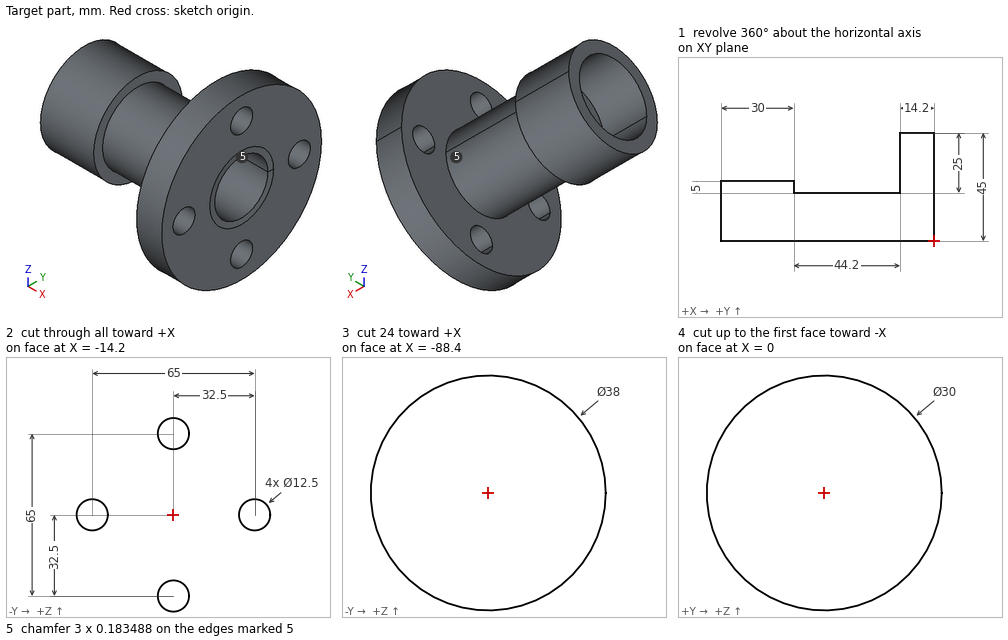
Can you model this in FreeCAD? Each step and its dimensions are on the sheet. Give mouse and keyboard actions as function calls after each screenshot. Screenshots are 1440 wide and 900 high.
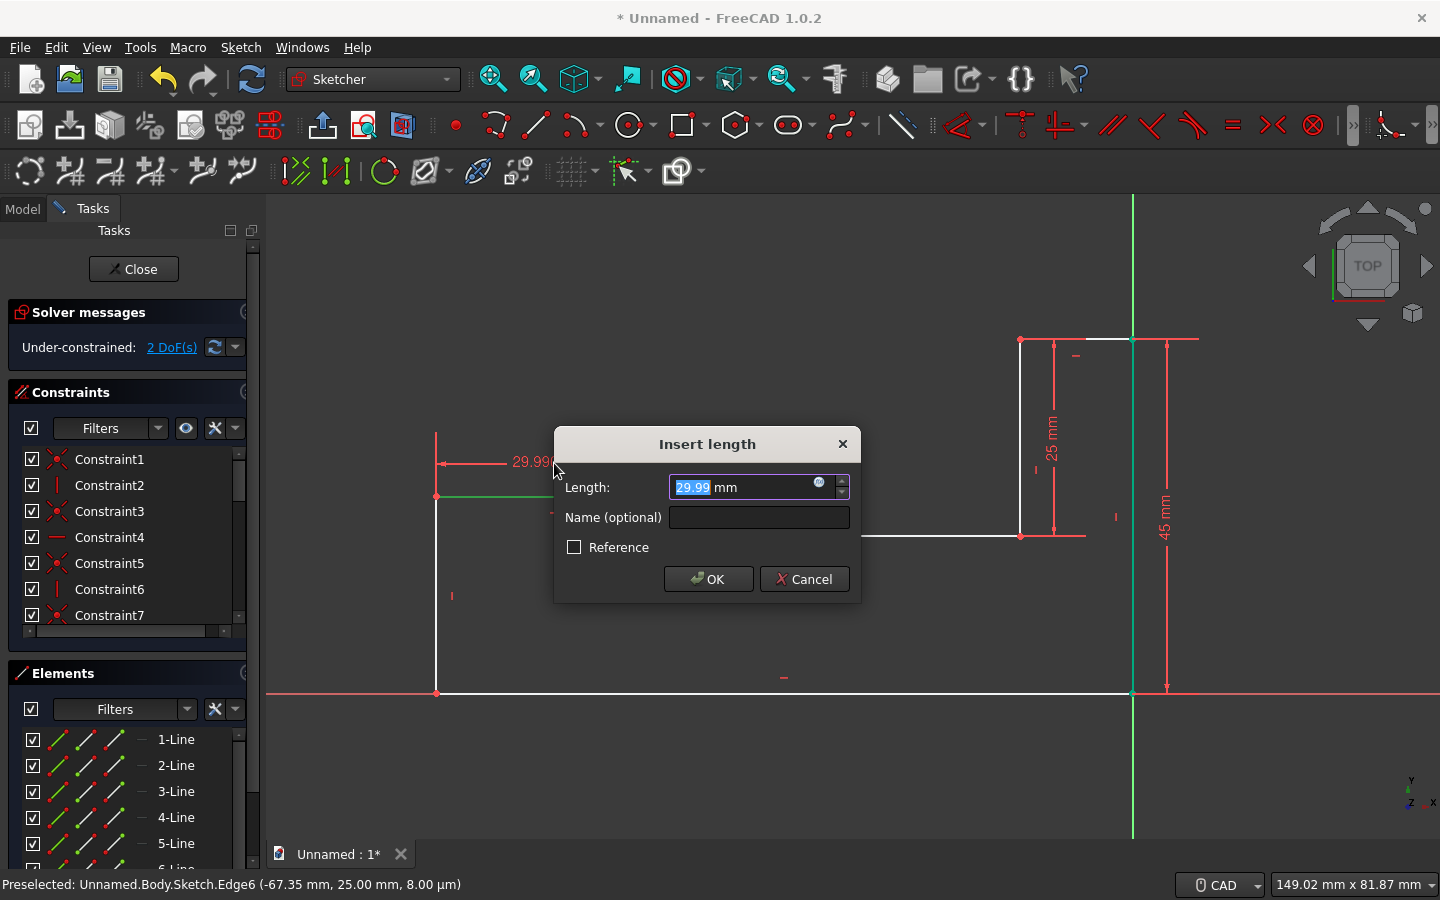
text(30)
key(Return)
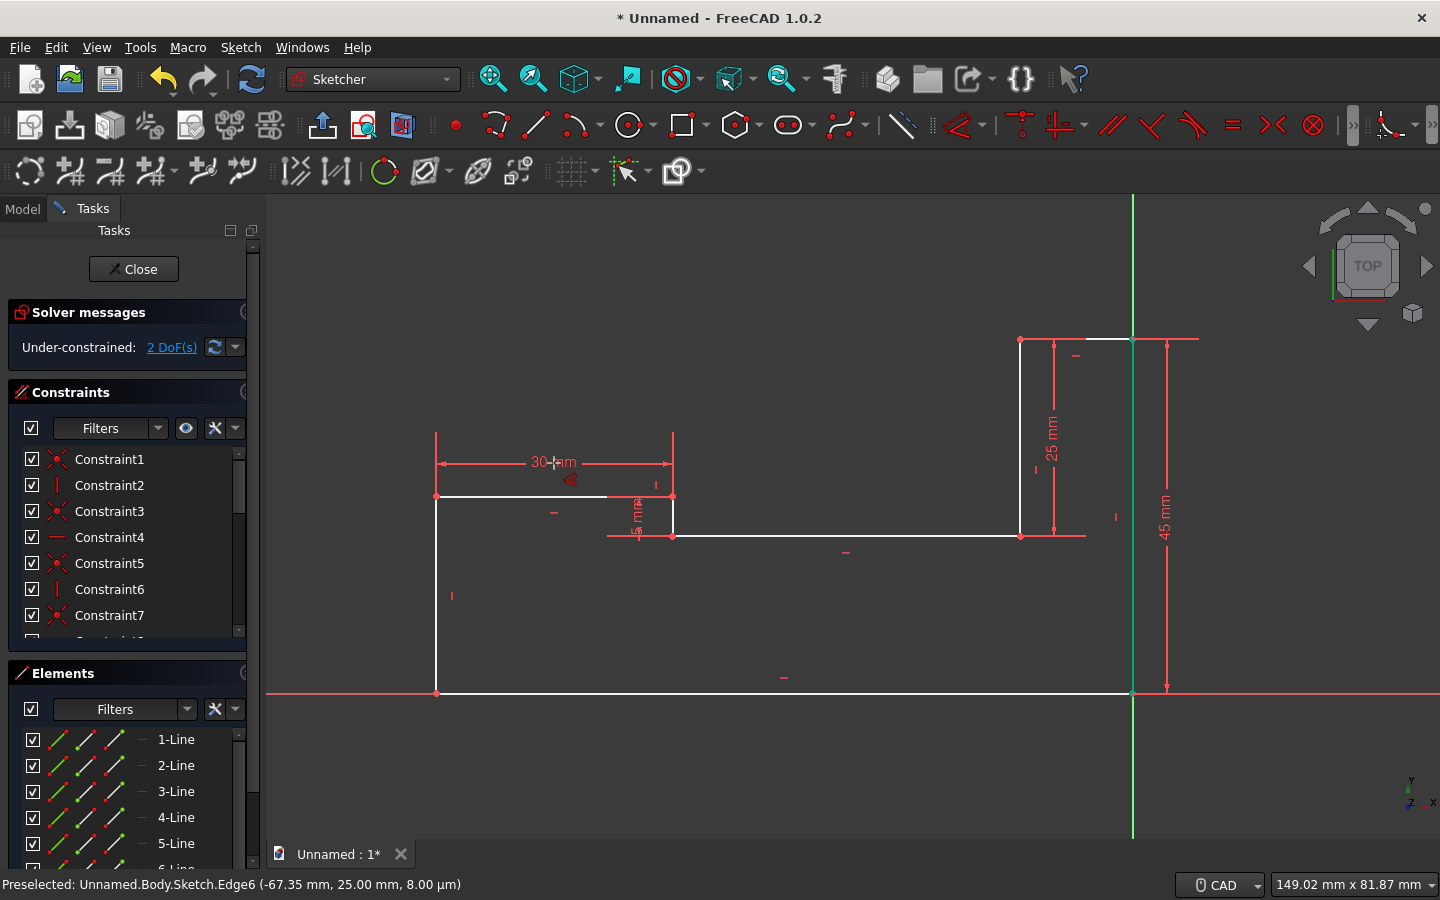
click(1099, 339)
click(1077, 305)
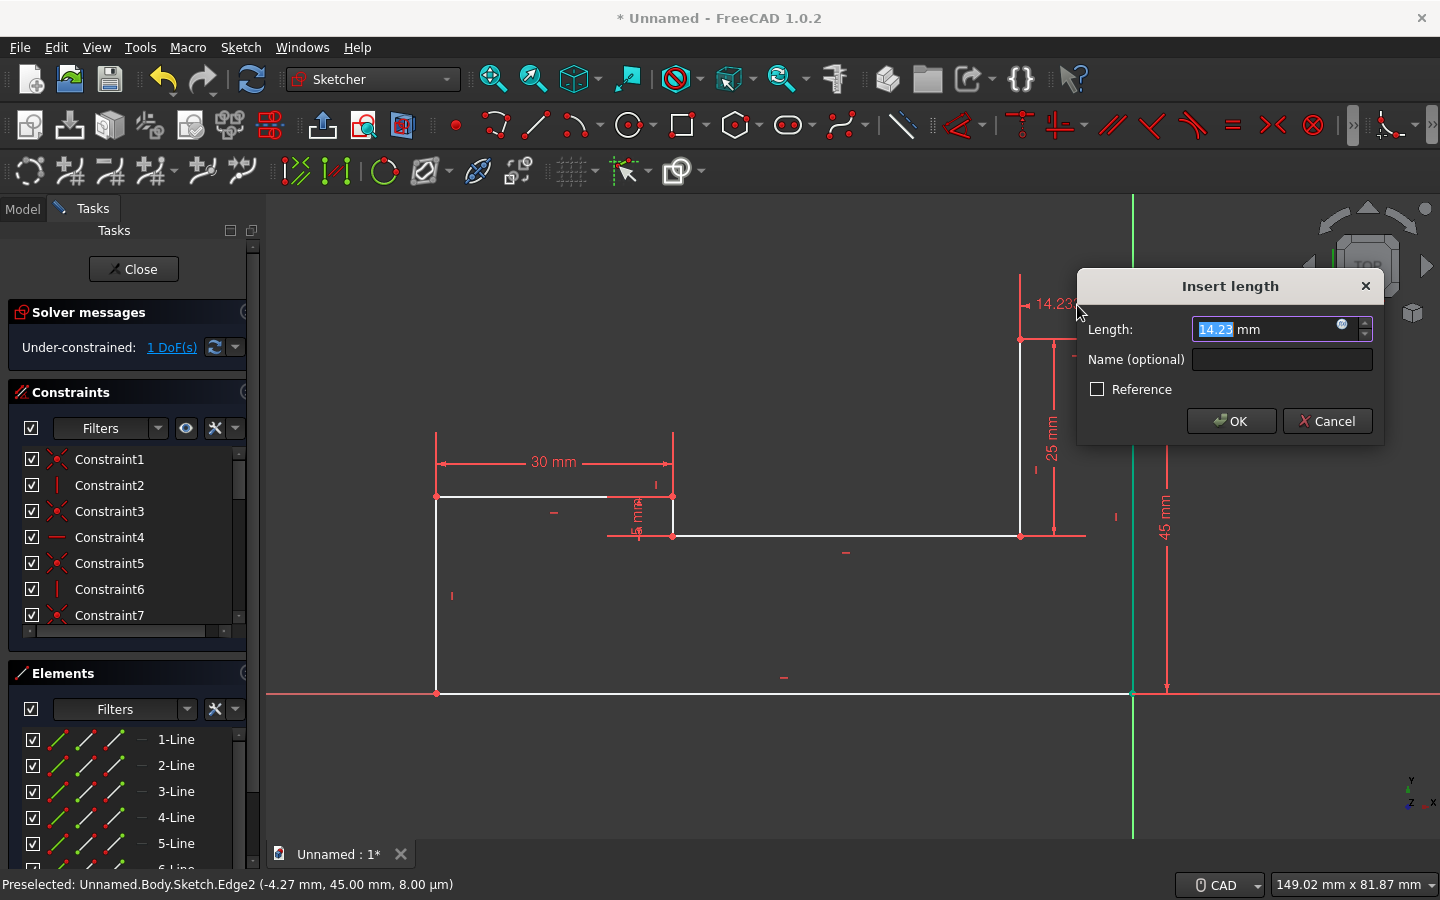
text(14.2)
key(Return)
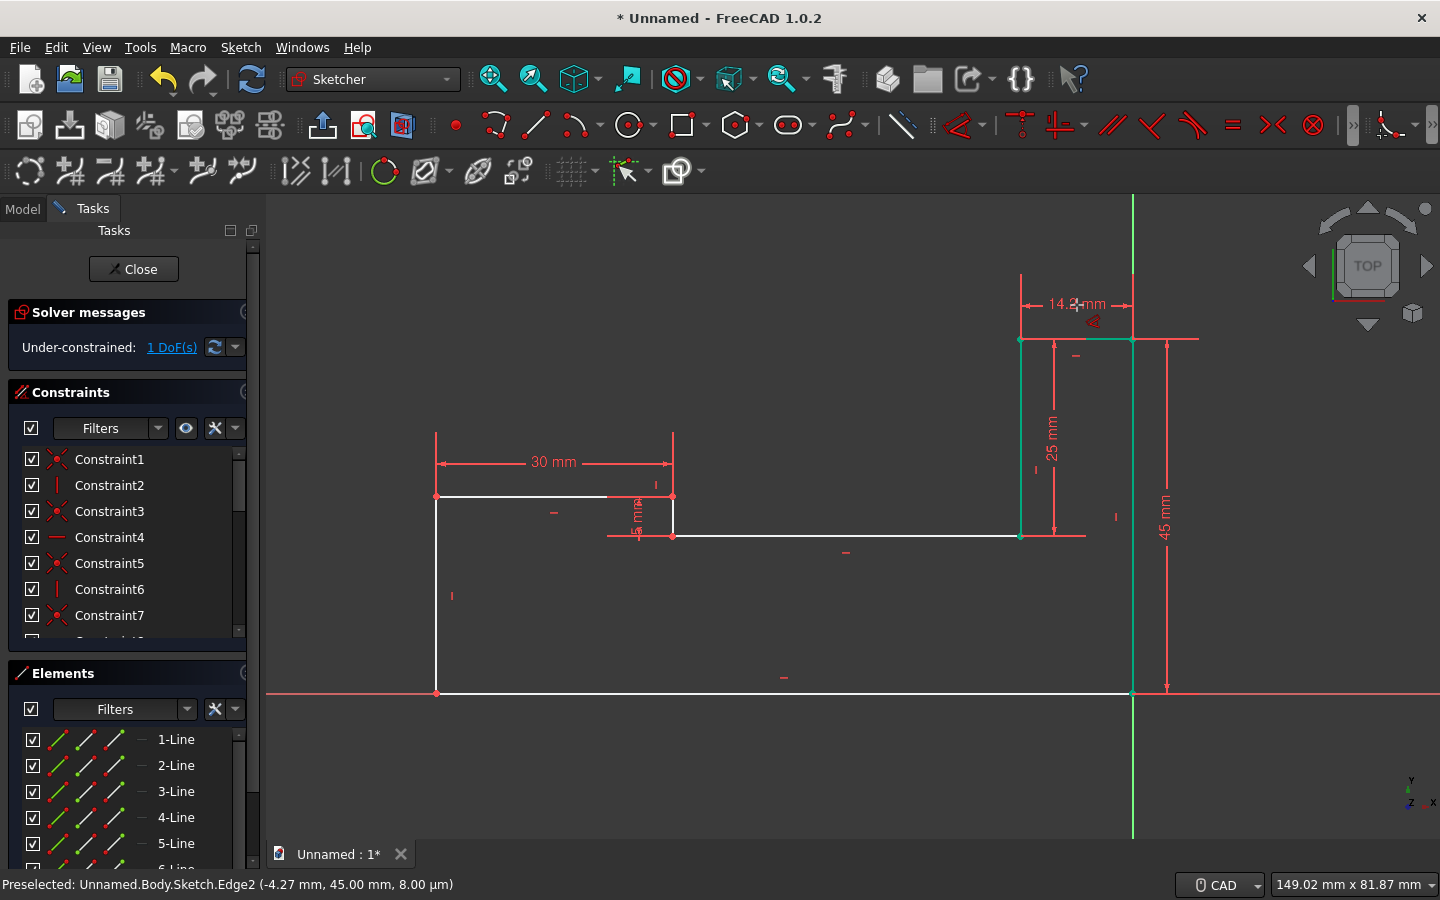
click(916, 536)
click(847, 570)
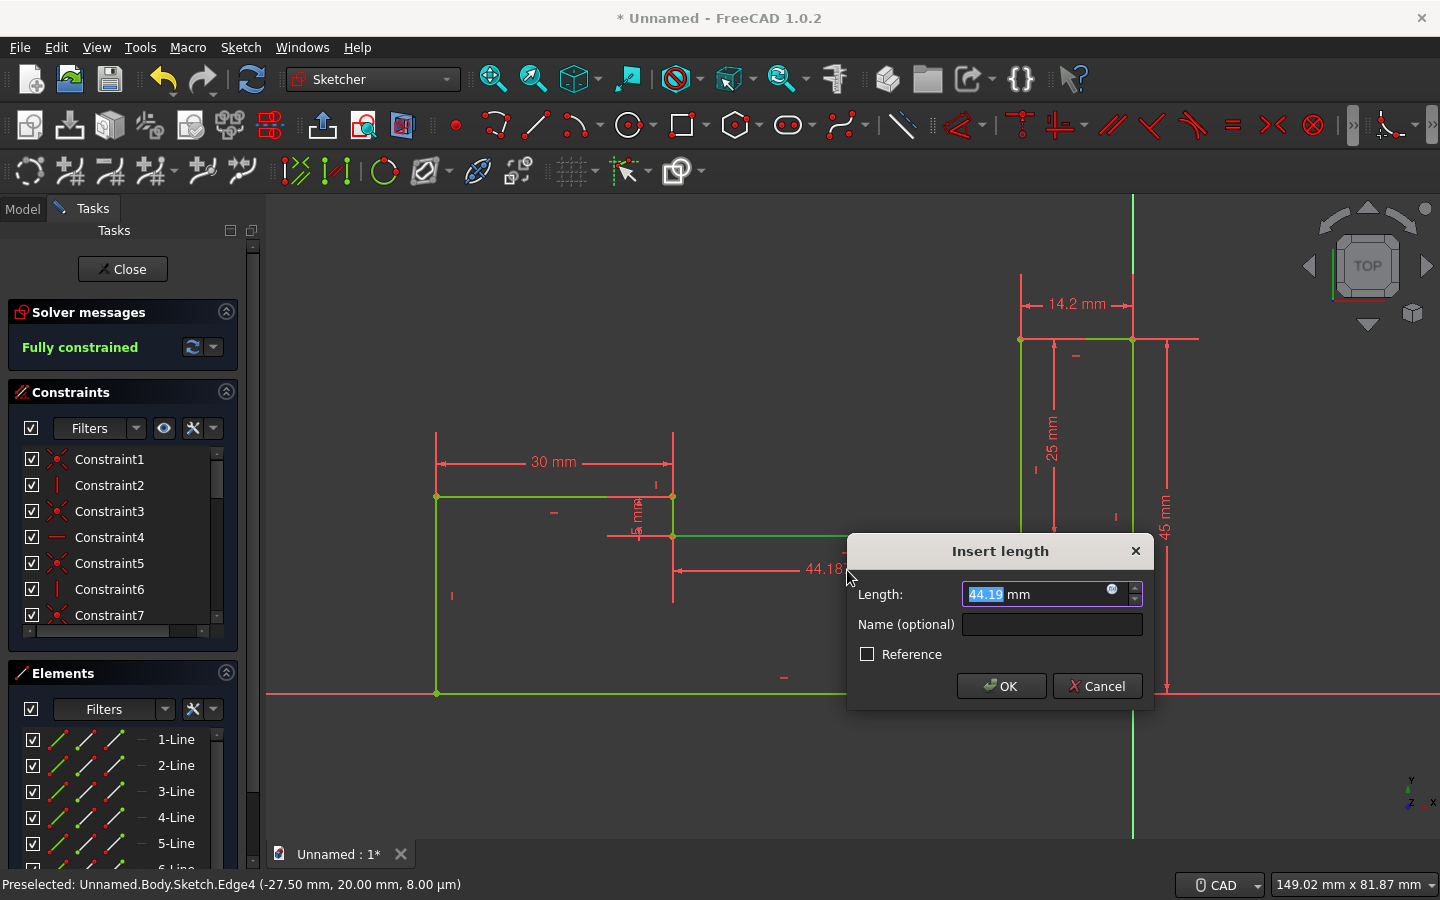
text(44.2)
key(Return)
key(Escape)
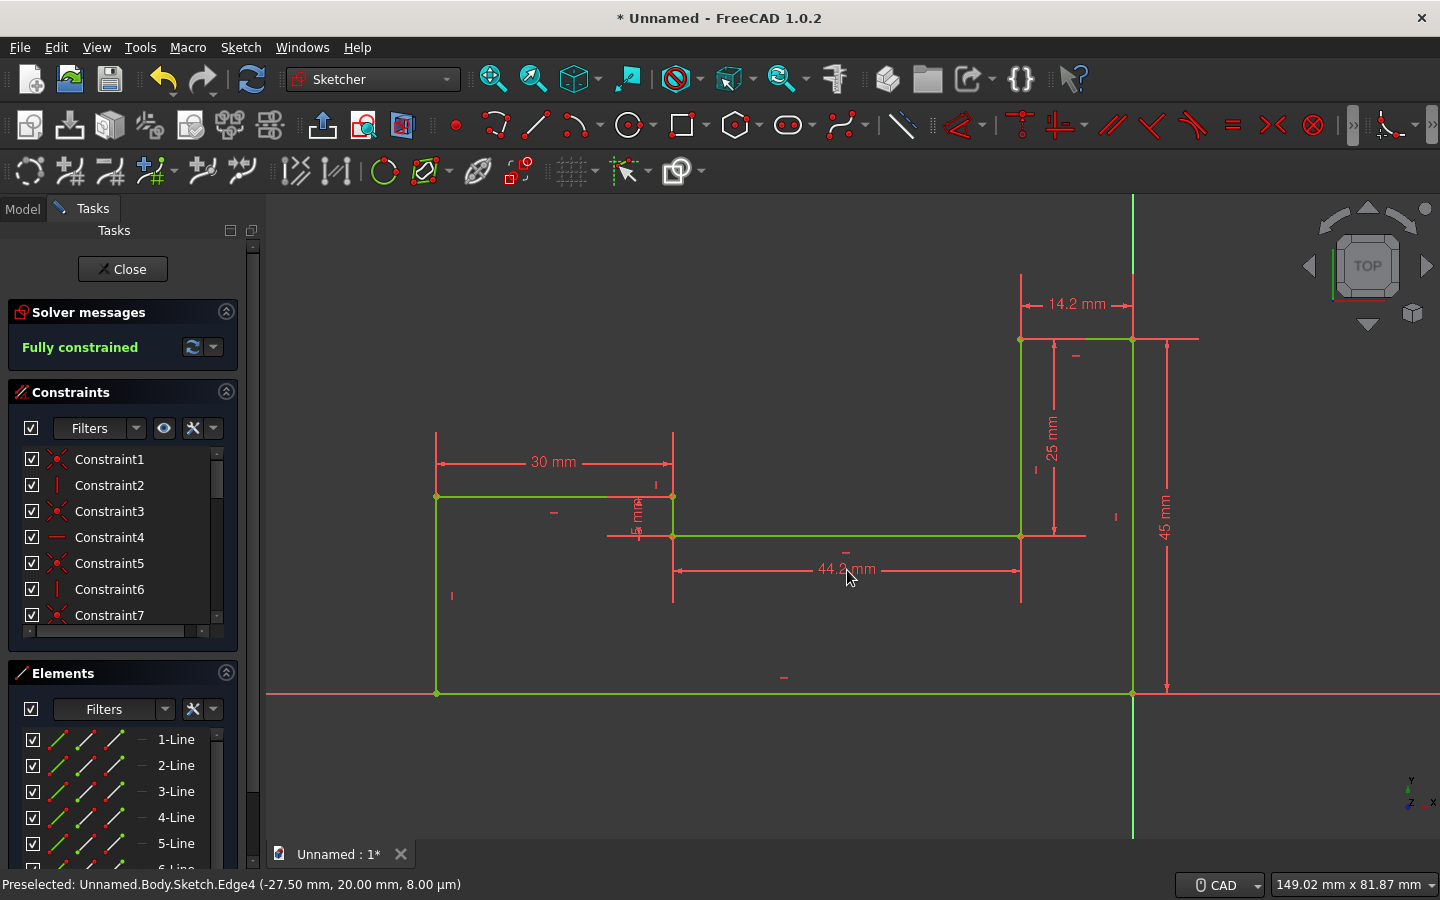
click(123, 269)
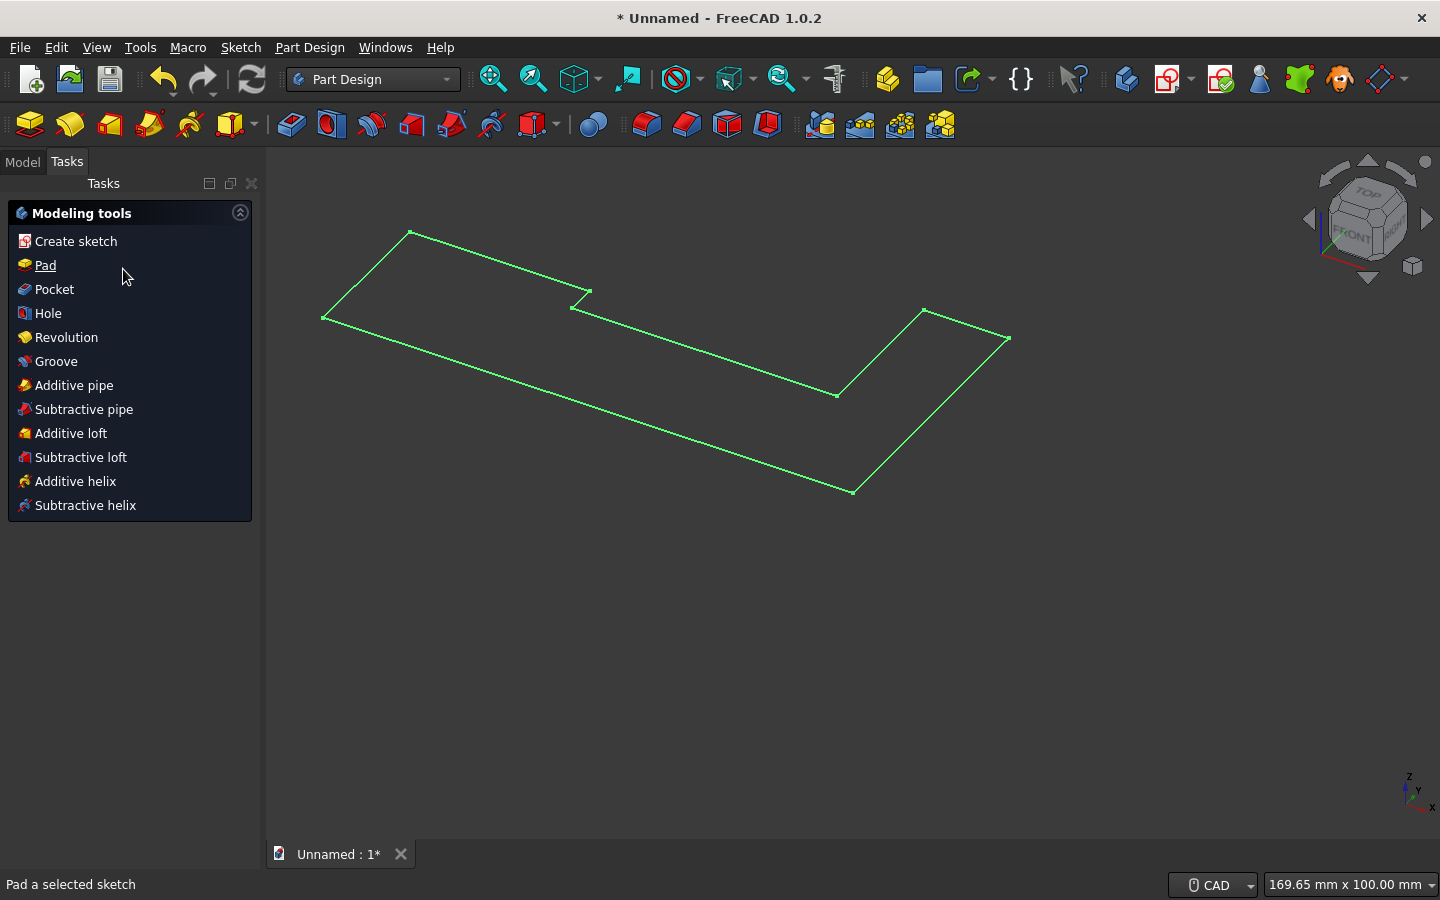
click(70, 124)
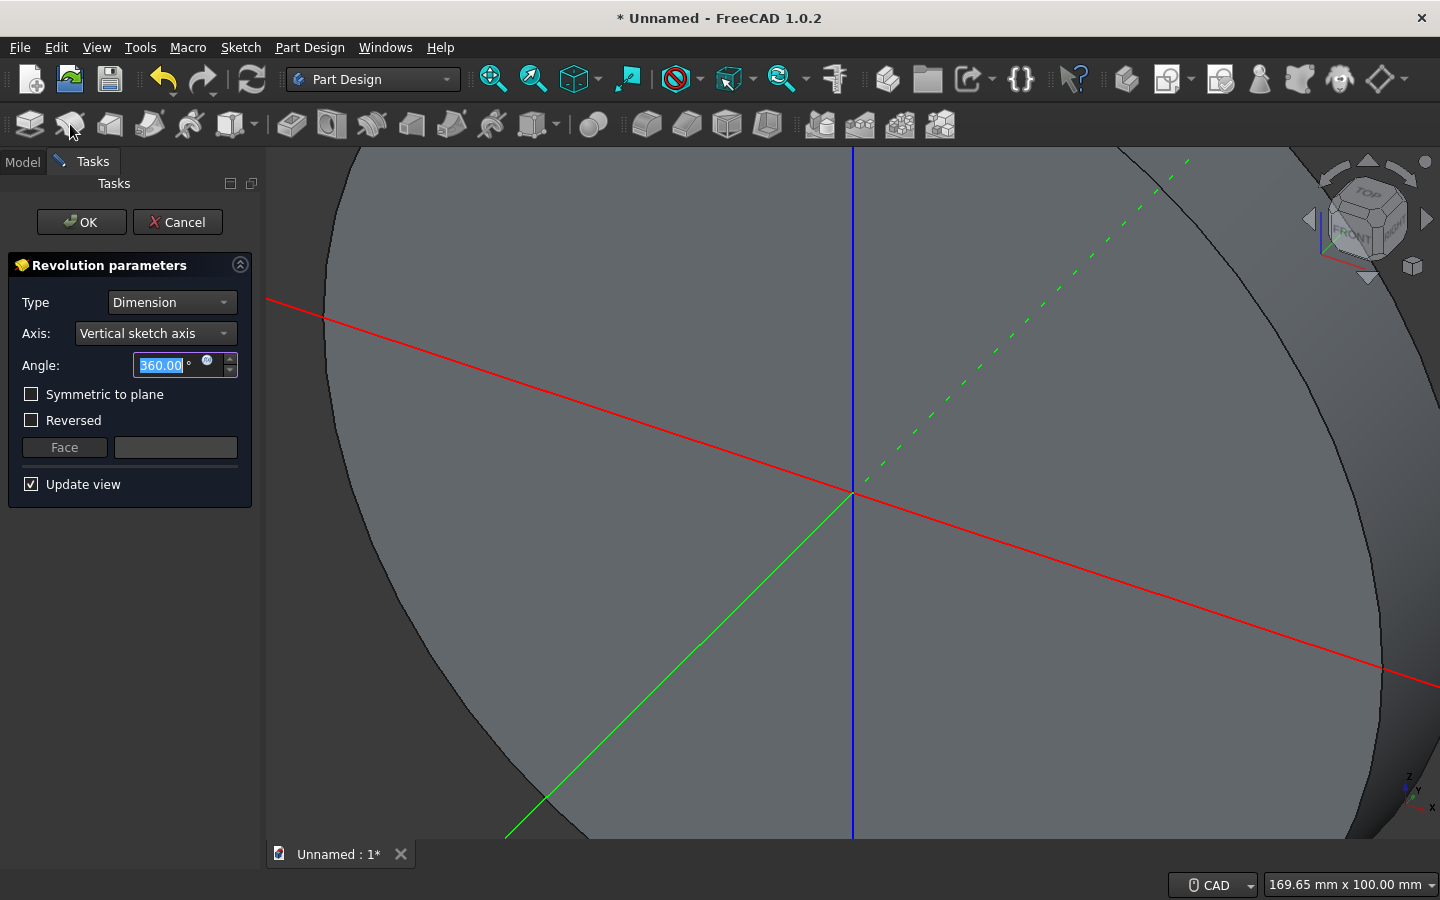
click(156, 334)